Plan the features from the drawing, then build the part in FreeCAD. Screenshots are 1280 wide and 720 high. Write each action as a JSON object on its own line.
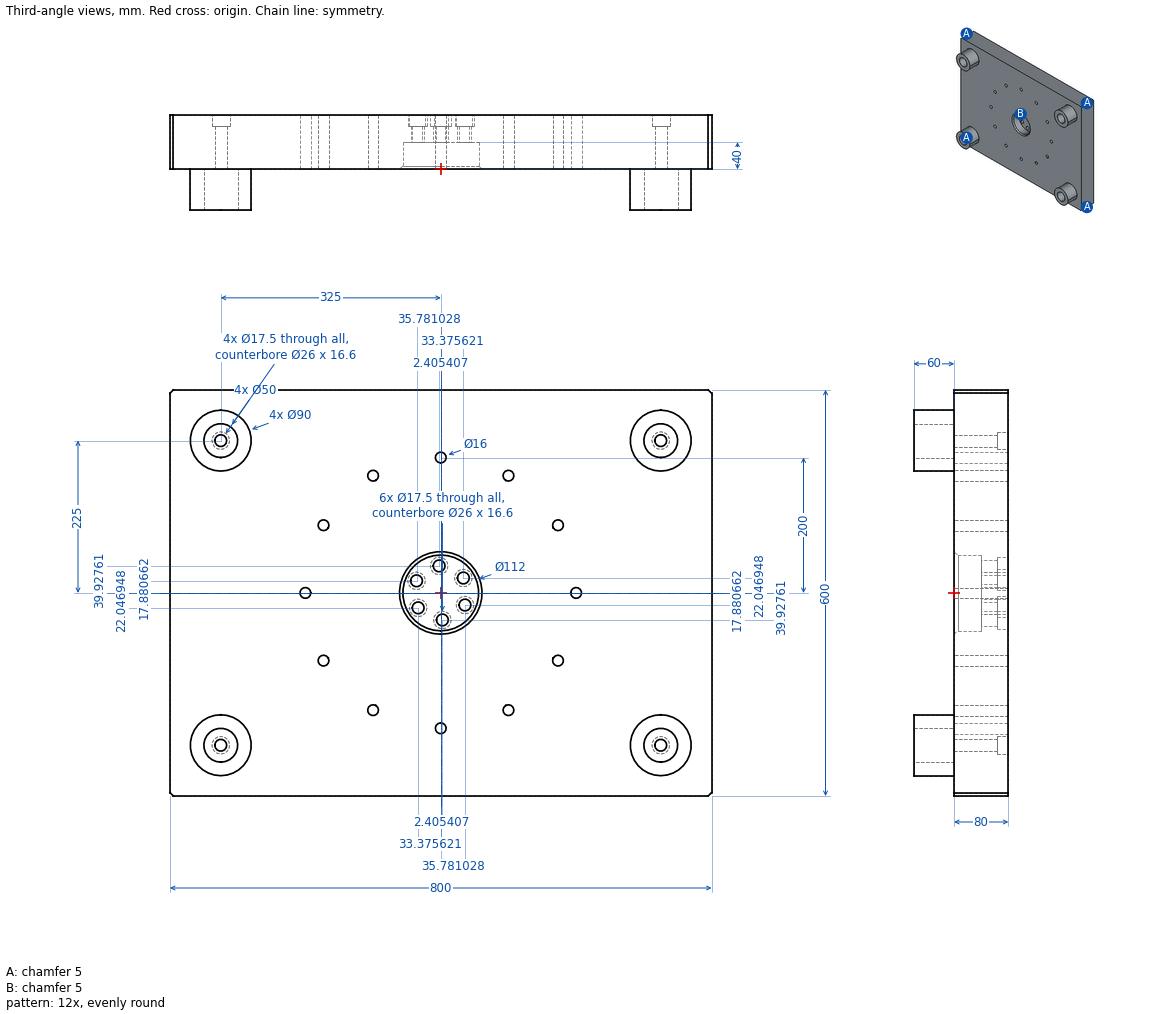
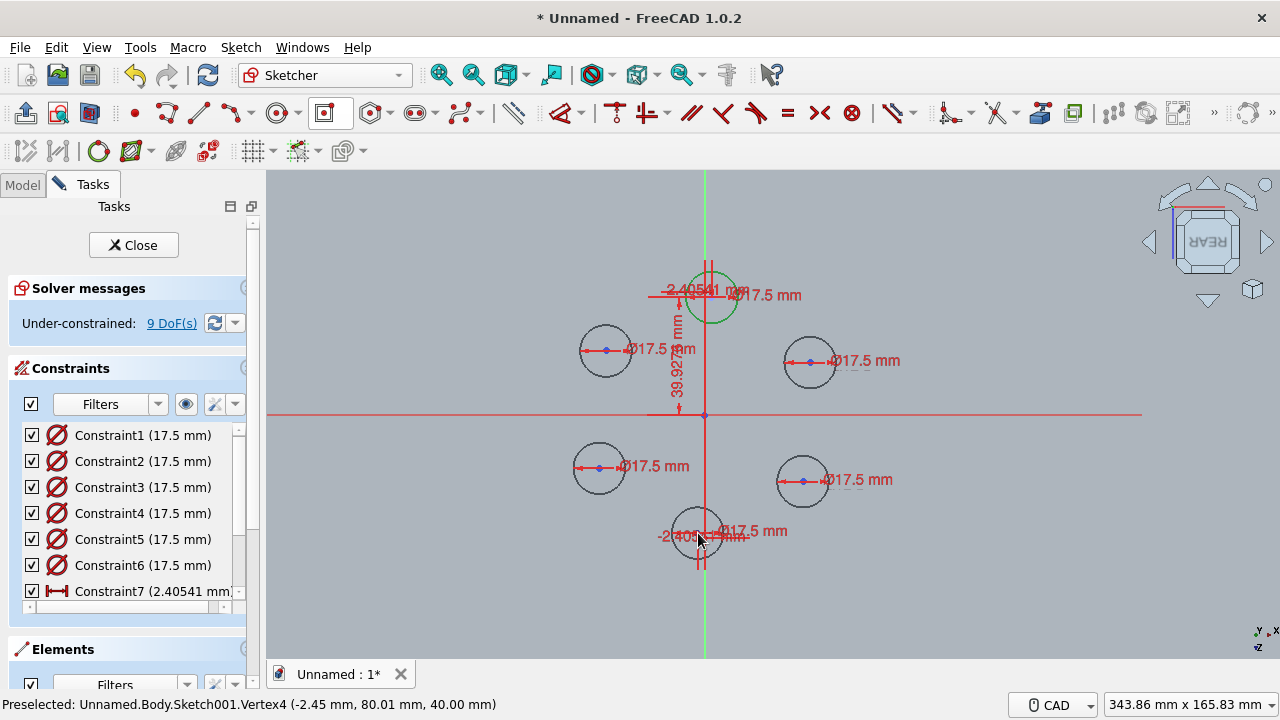
{"action": "left_click", "coordinate": [698, 533]}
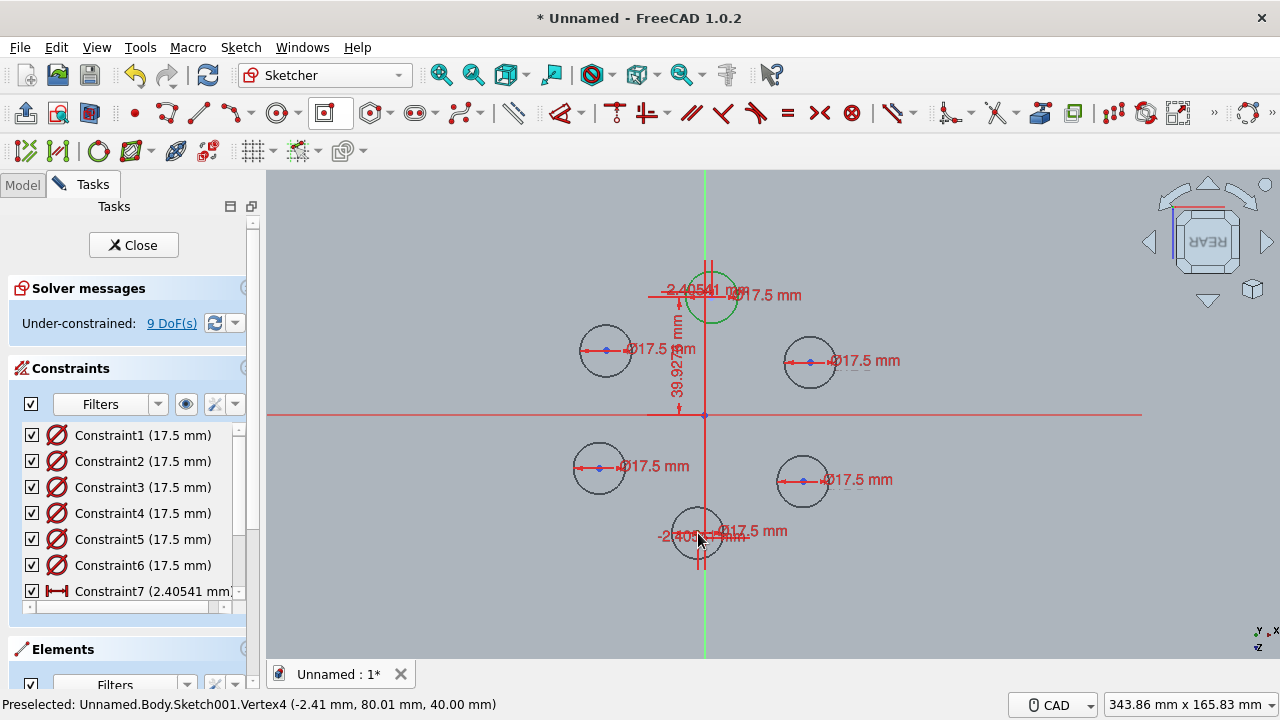
{"action": "key", "text": "i"}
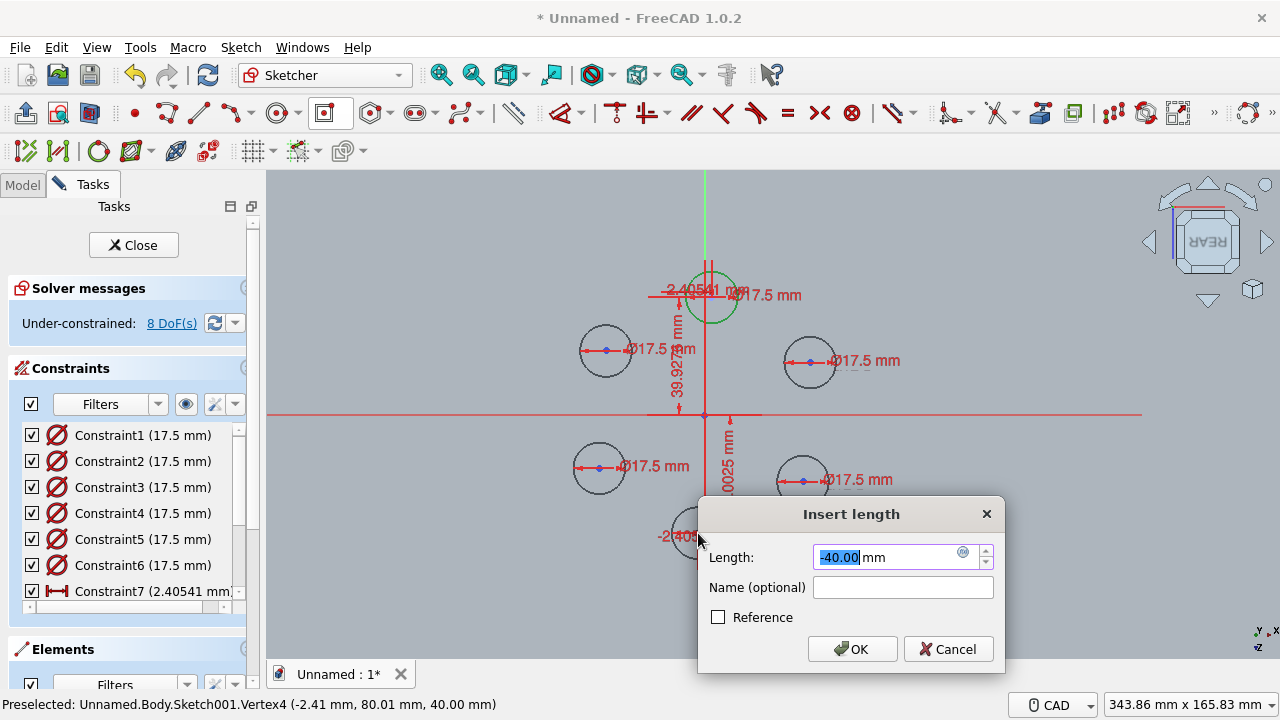
{"action": "type", "text": "-39.92761"}
{"action": "key", "text": "Return"}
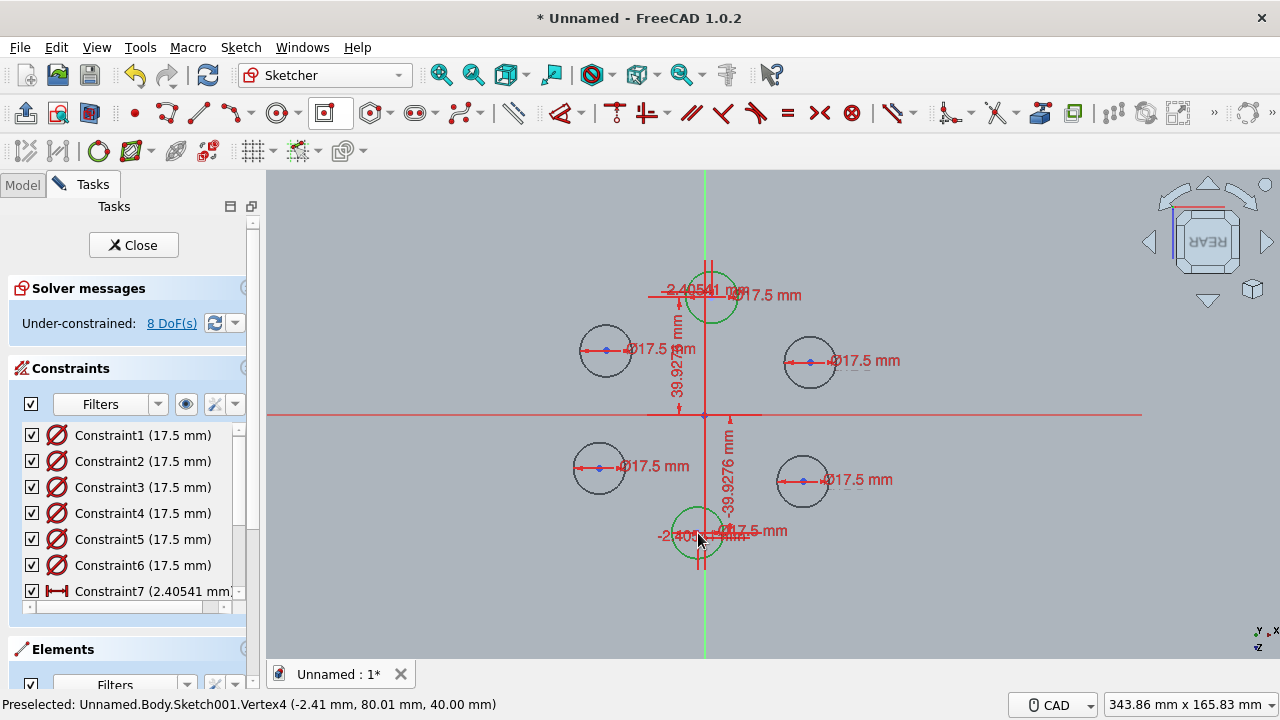
{"action": "left_click", "coordinate": [810, 363]}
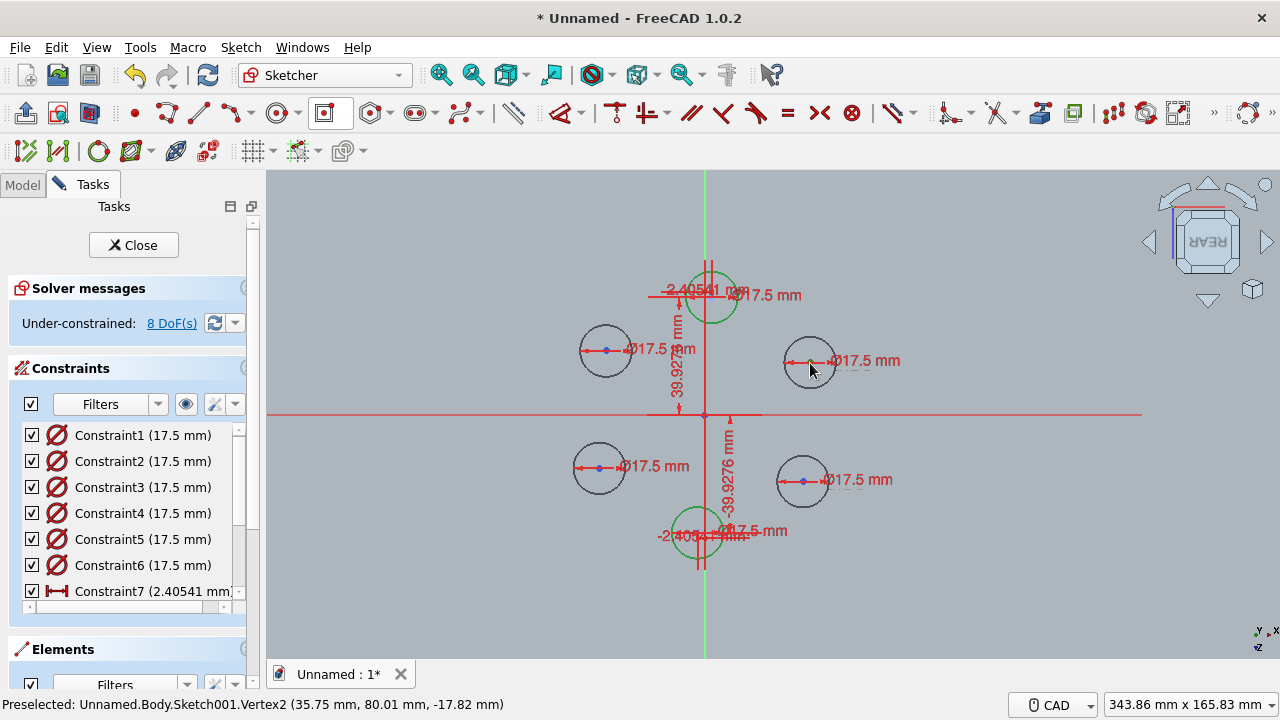
{"action": "key", "text": "l"}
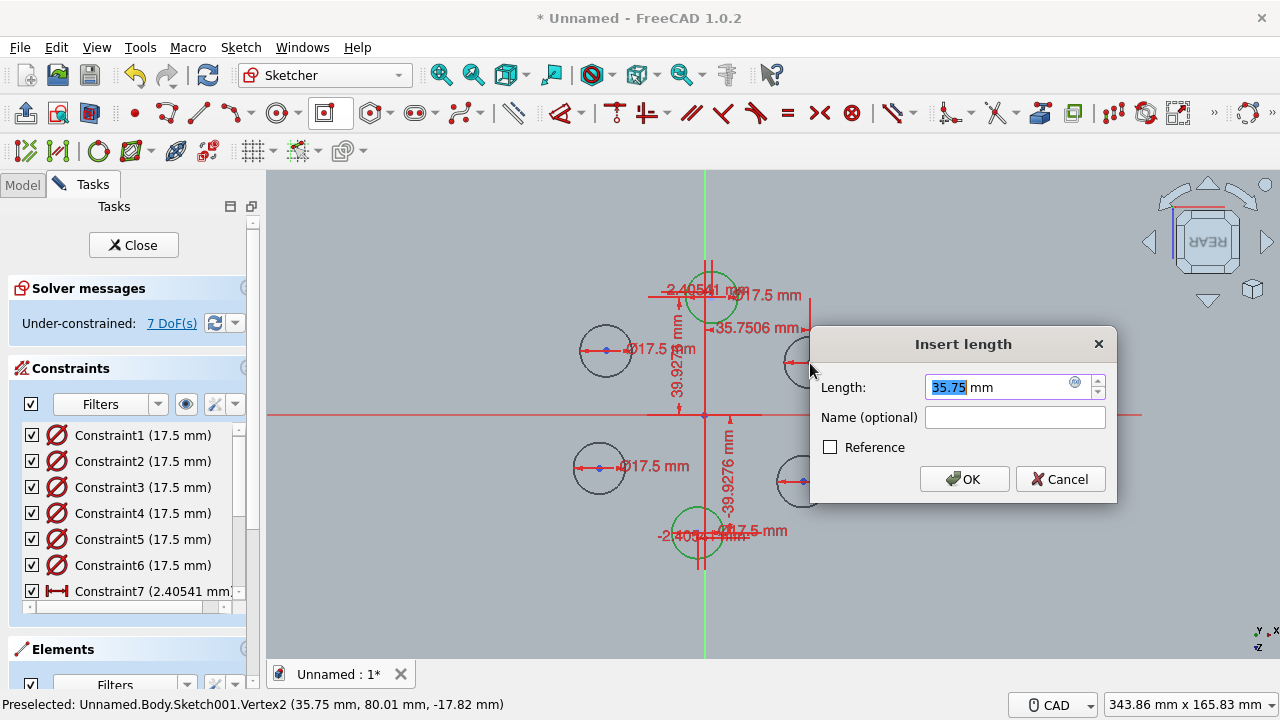
{"action": "type", "text": "35.781028"}
{"action": "key", "text": "Return"}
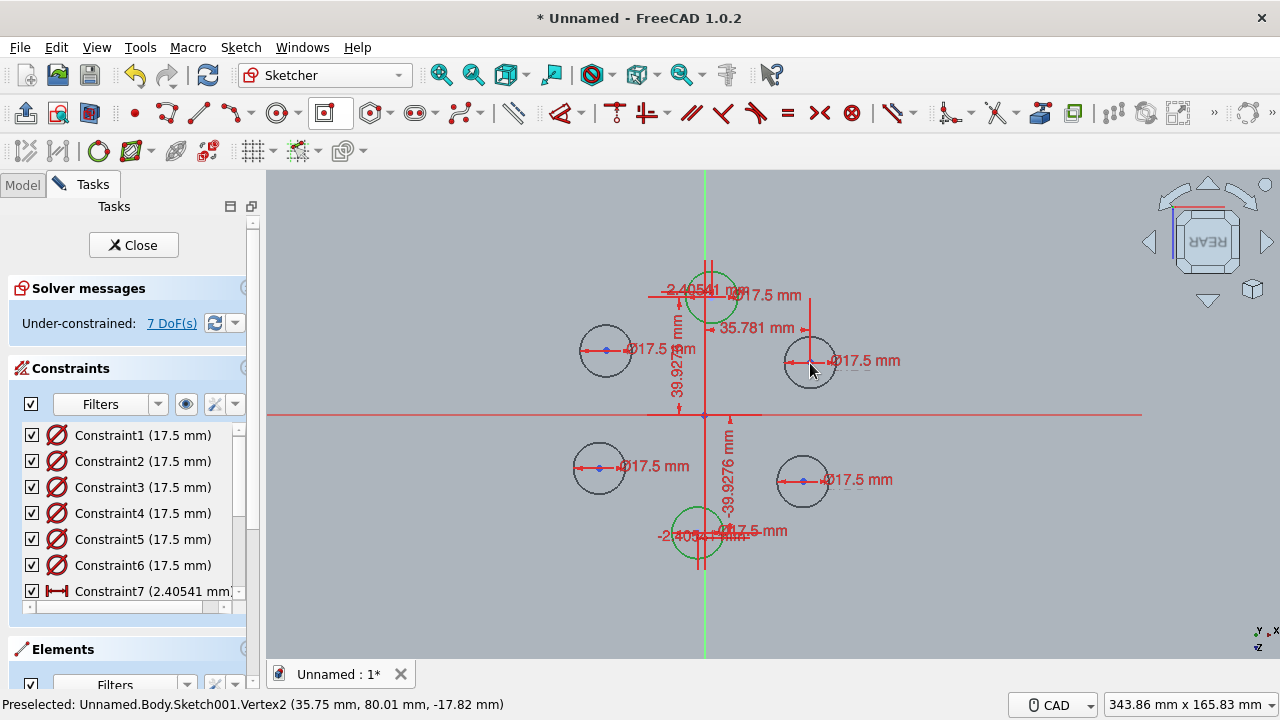
{"action": "left_click", "coordinate": [810, 363]}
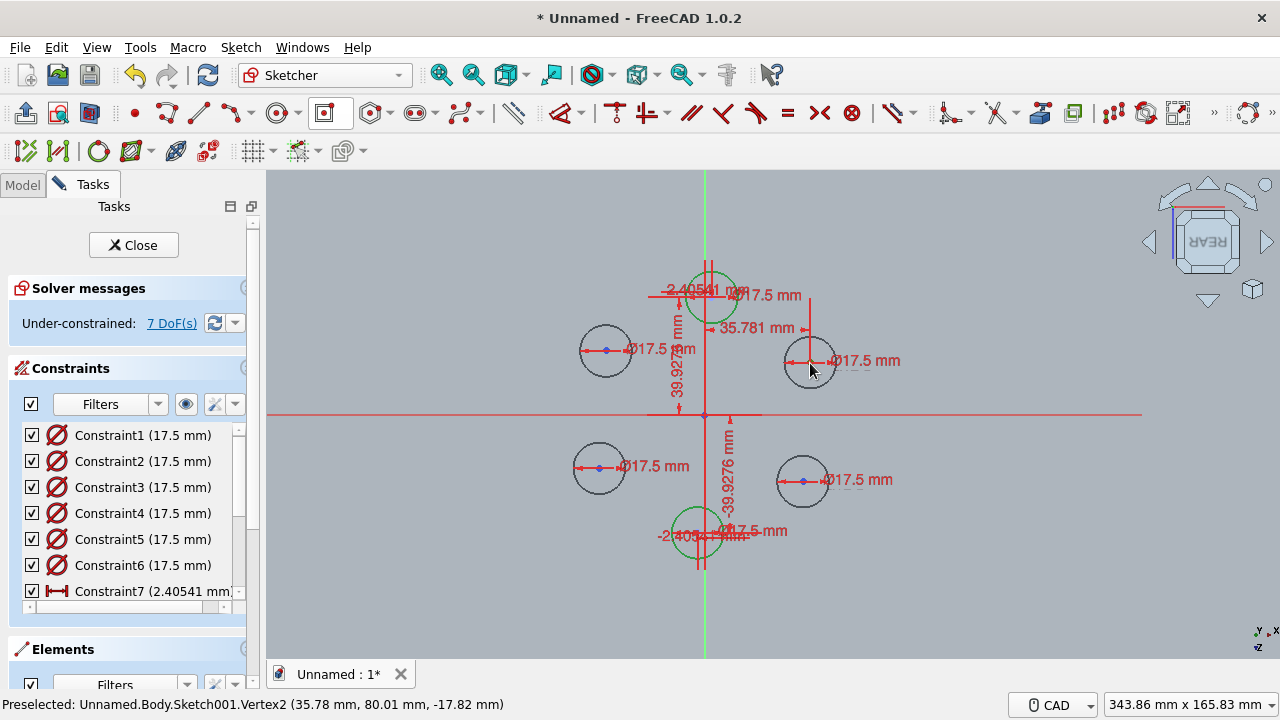
{"action": "key", "text": "i"}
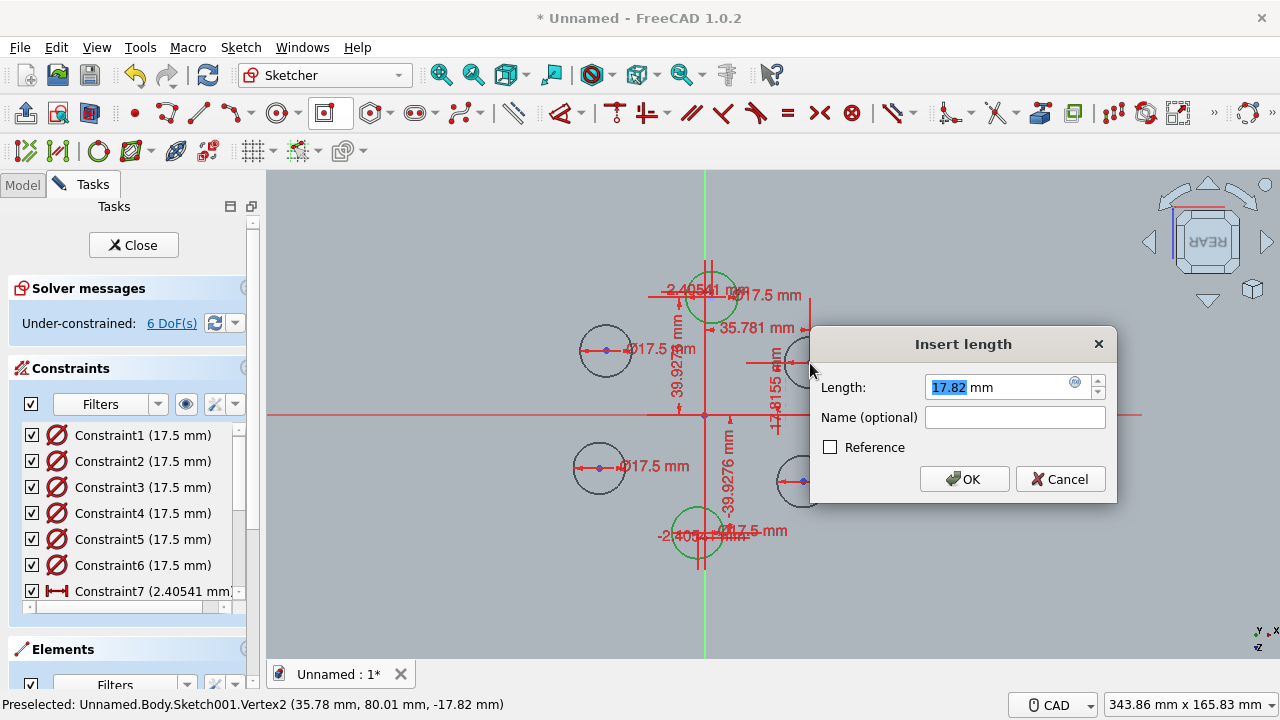
{"action": "type", "text": "17.880662"}
{"action": "key", "text": "Return"}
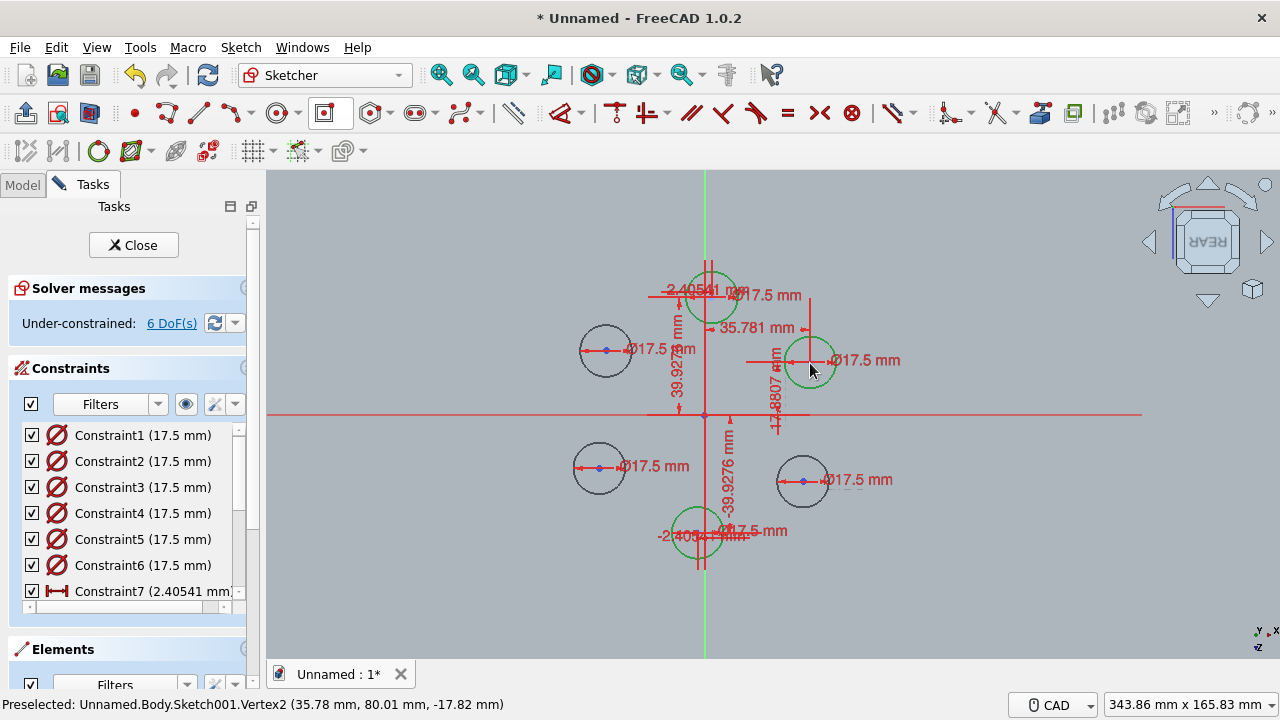
{"action": "left_click", "coordinate": [803, 482]}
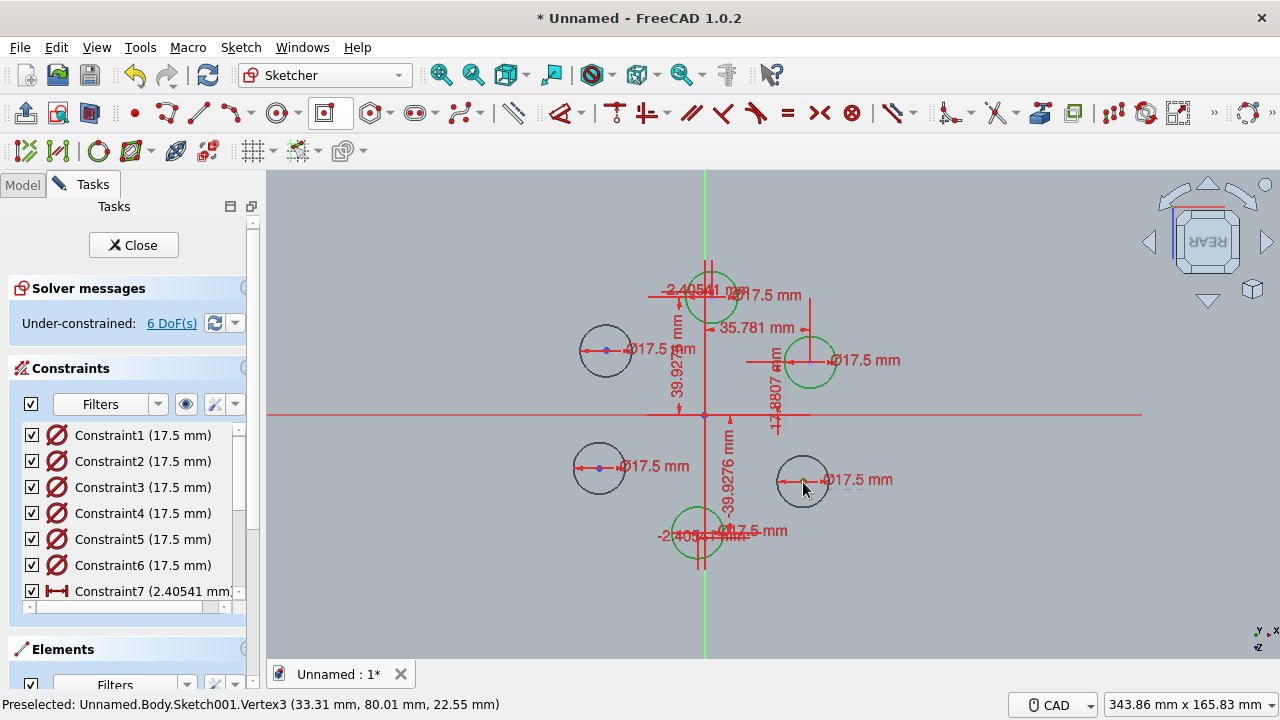
{"action": "key", "text": "l"}